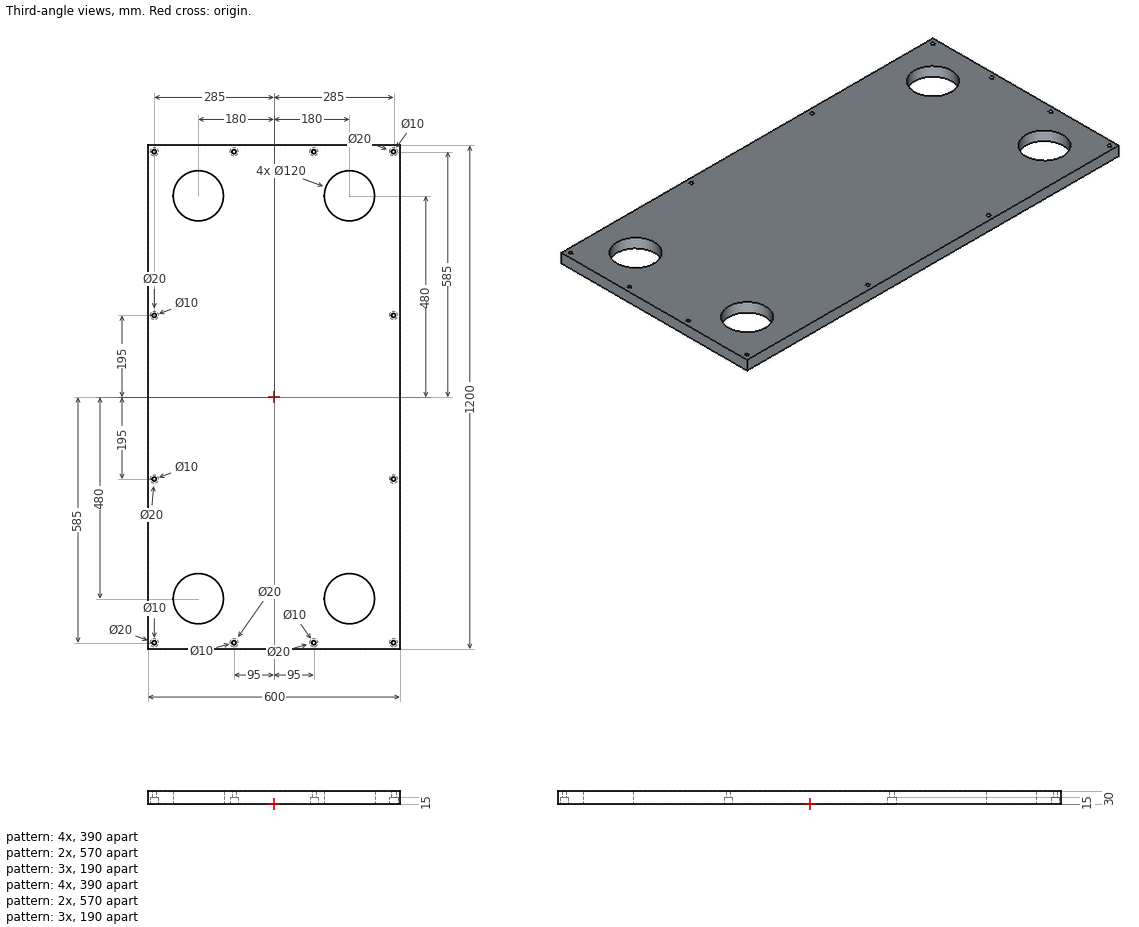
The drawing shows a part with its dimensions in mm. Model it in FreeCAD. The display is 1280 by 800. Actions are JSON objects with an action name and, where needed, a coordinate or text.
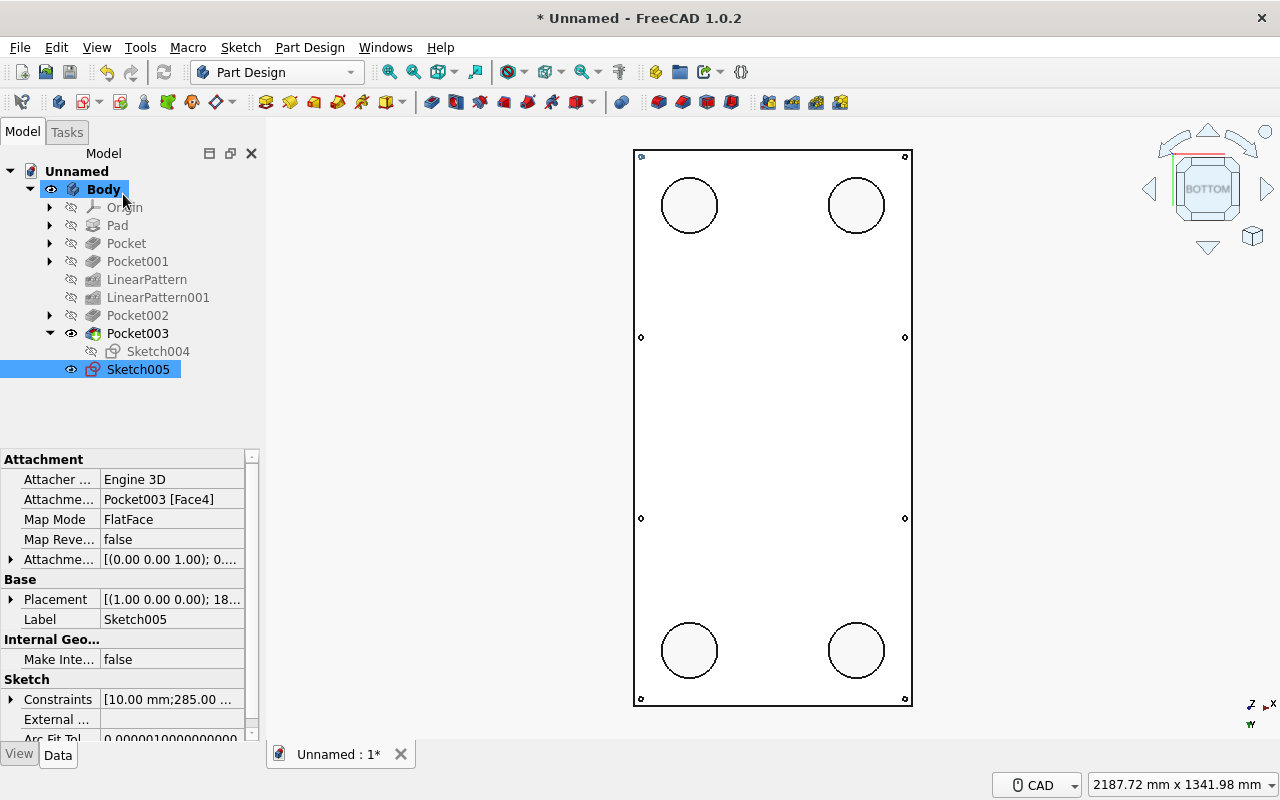
{"action": "left_click", "coordinate": [432, 102]}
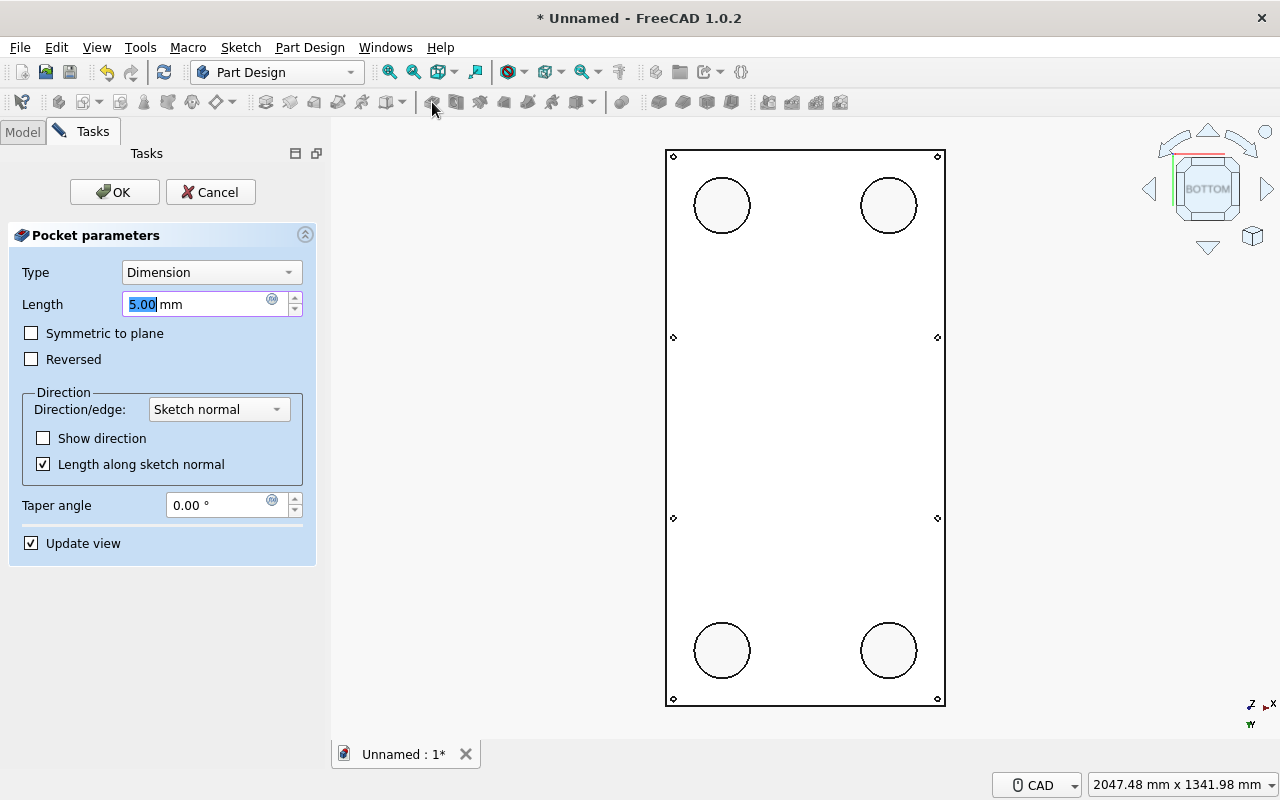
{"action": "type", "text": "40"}
{"action": "key", "text": "Tab"}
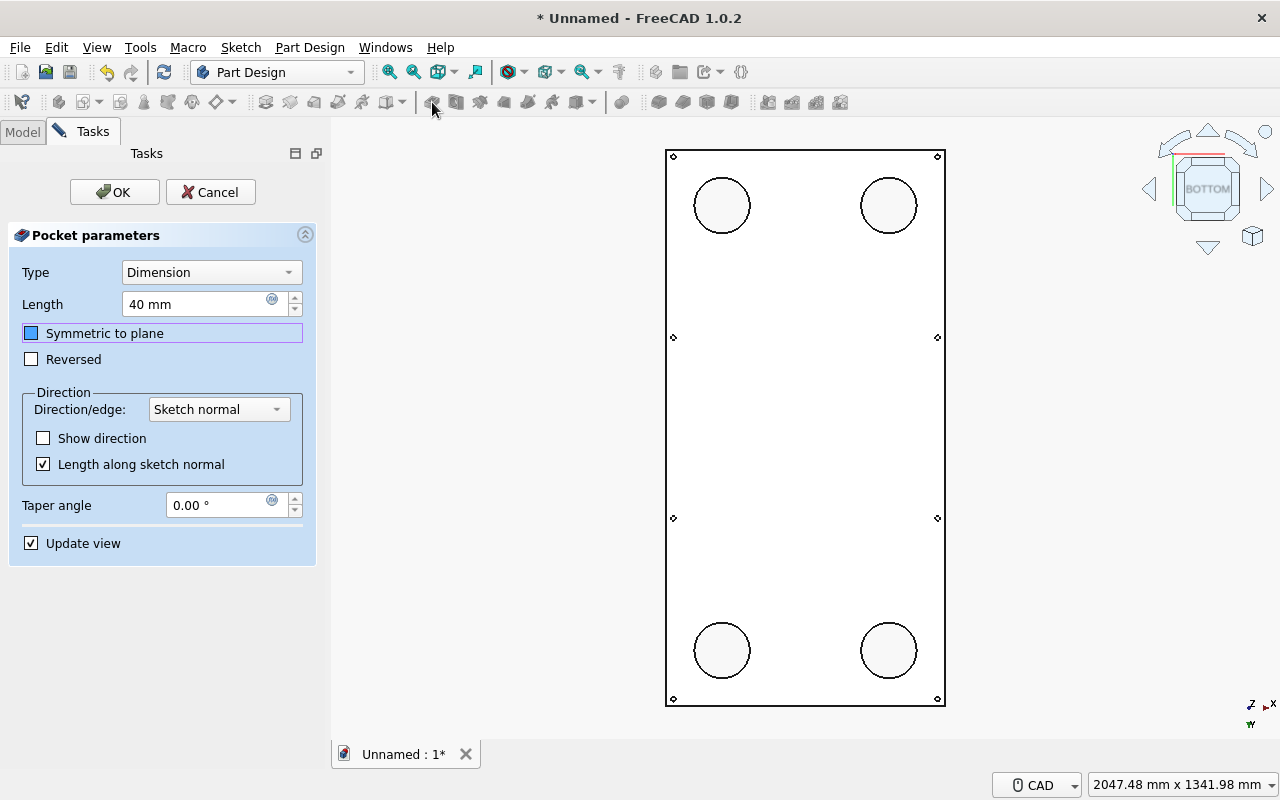
{"action": "left_click", "coordinate": [115, 192]}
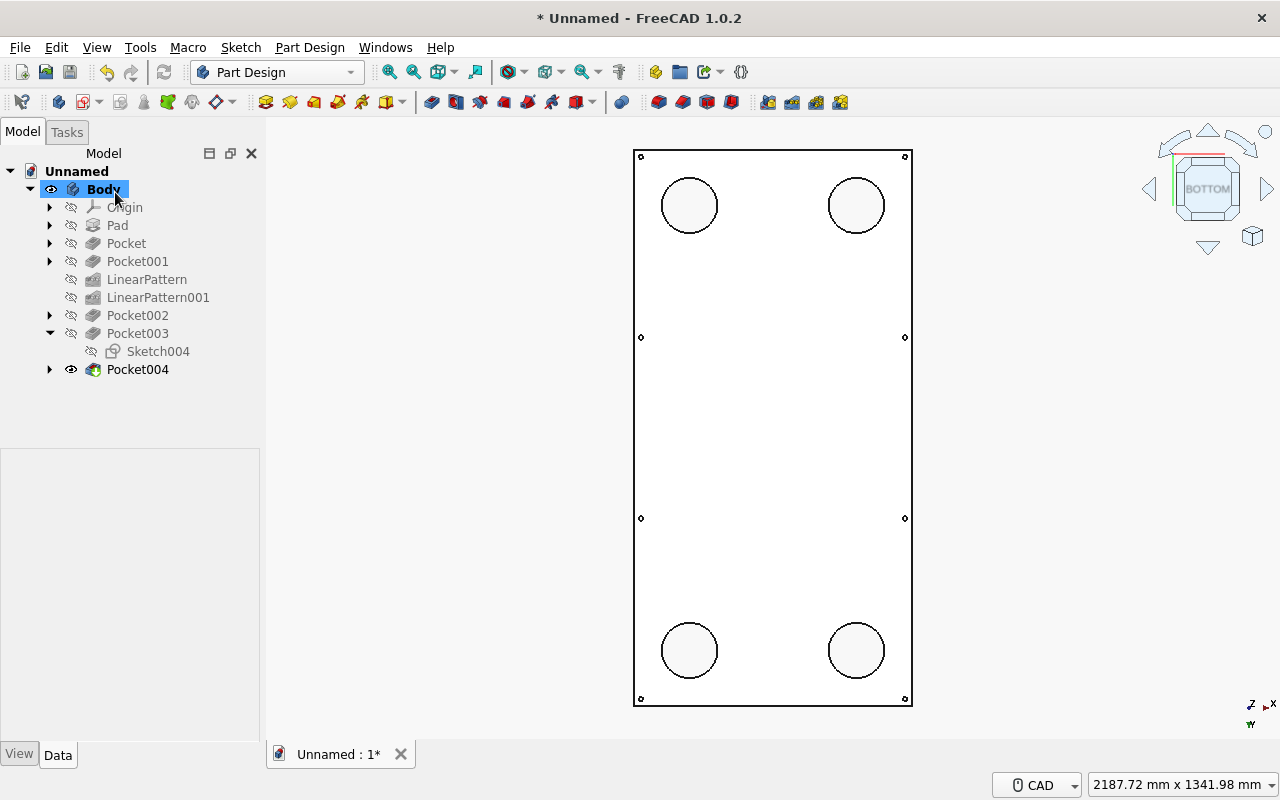
{"action": "left_click", "coordinate": [116, 261]}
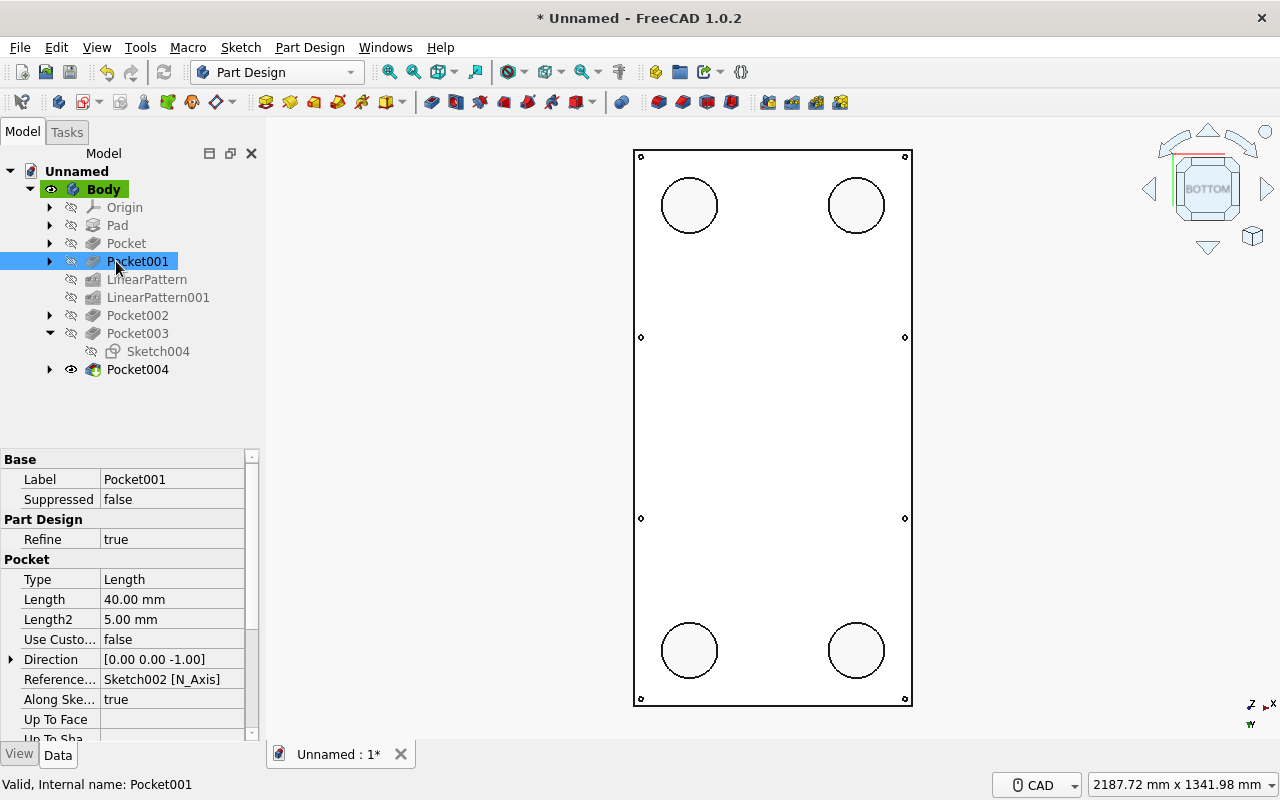
{"action": "left_click", "coordinate": [792, 102]}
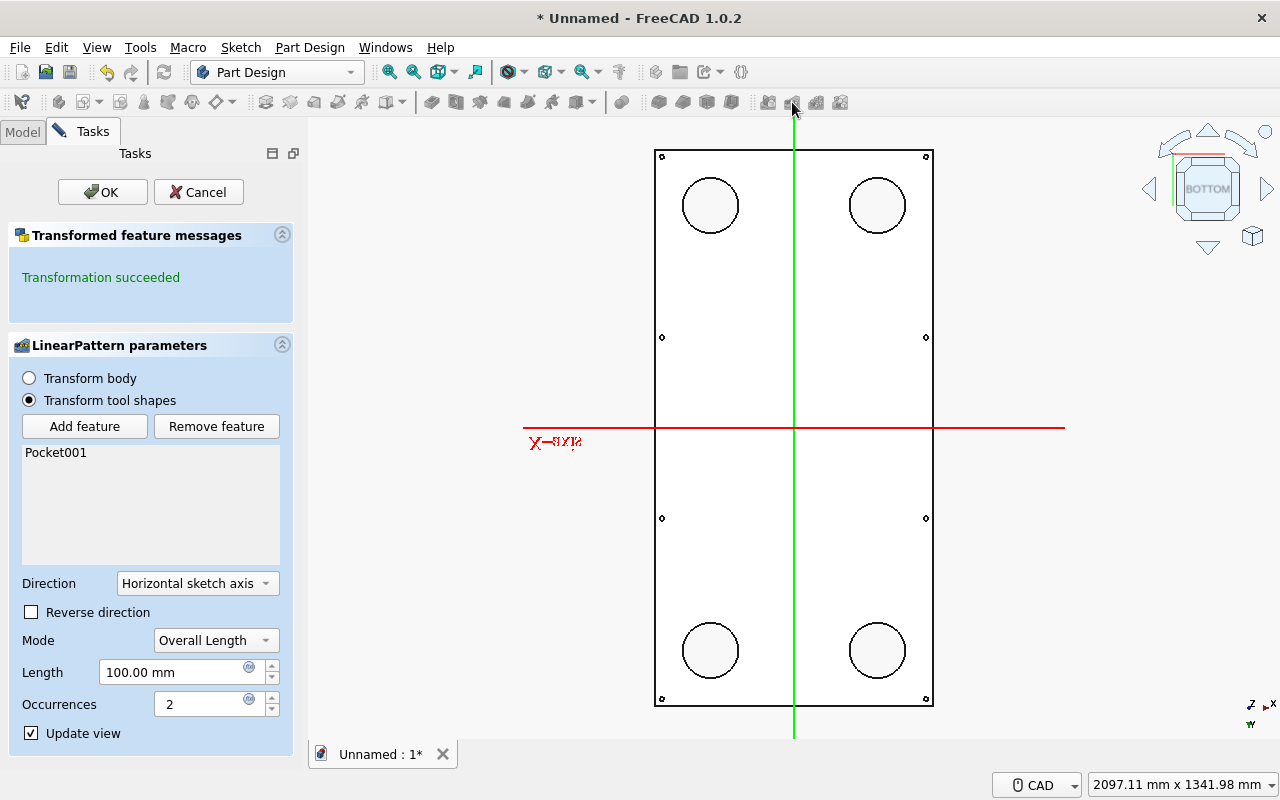
{"action": "left_click", "coordinate": [198, 584]}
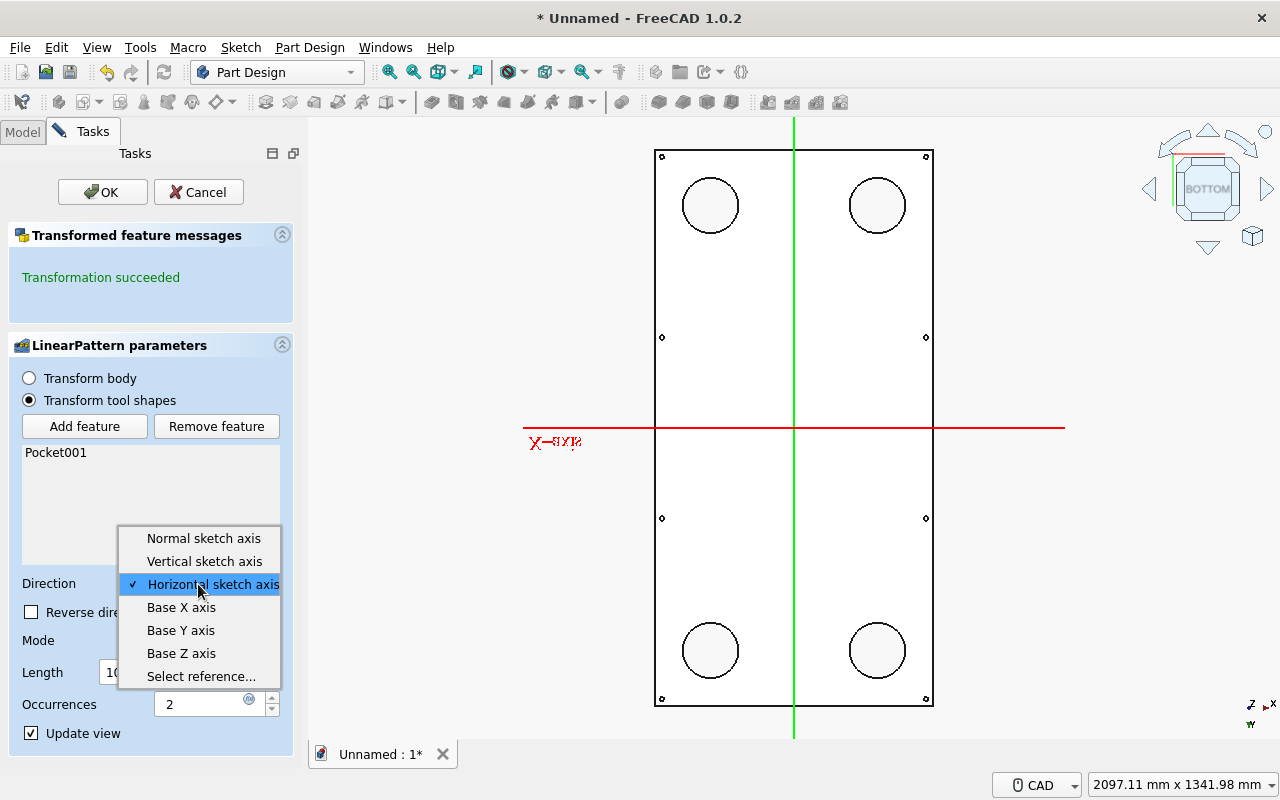
{"action": "left_click", "coordinate": [198, 608]}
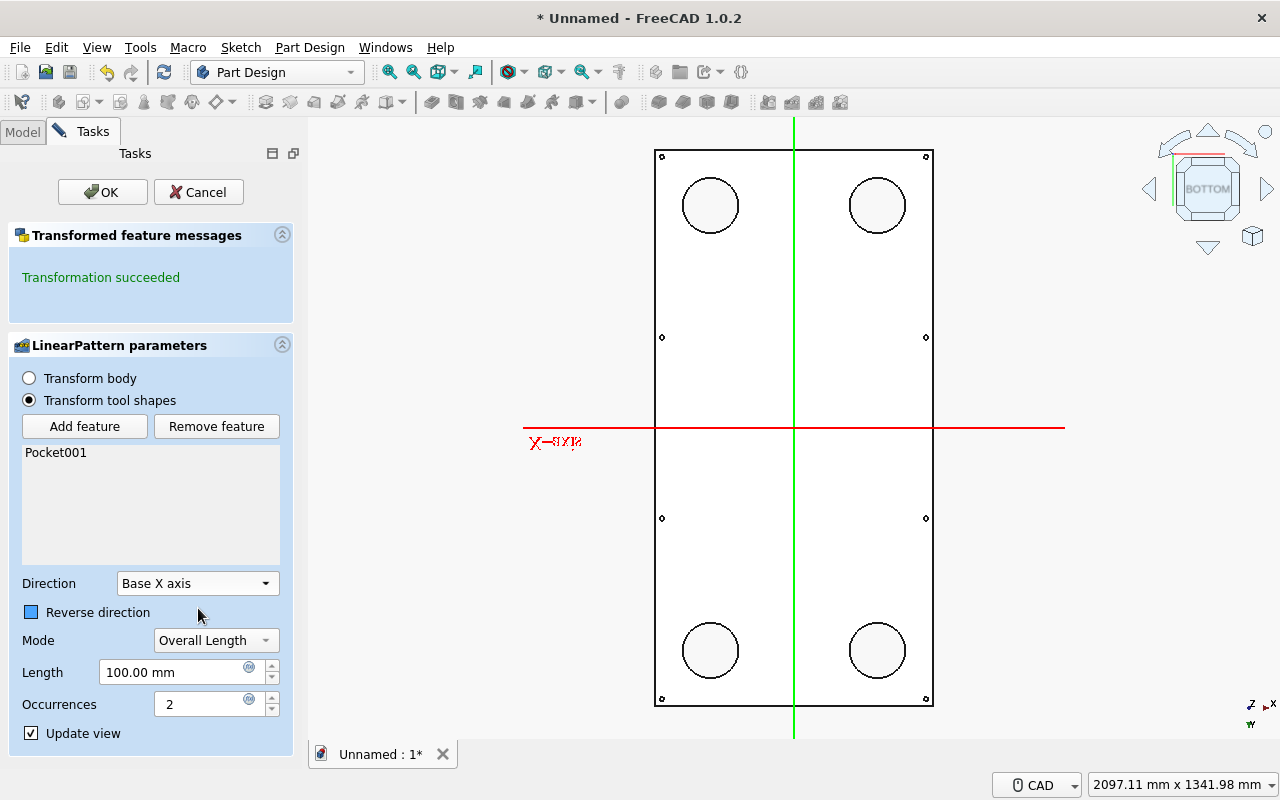
{"action": "left_click", "coordinate": [217, 640]}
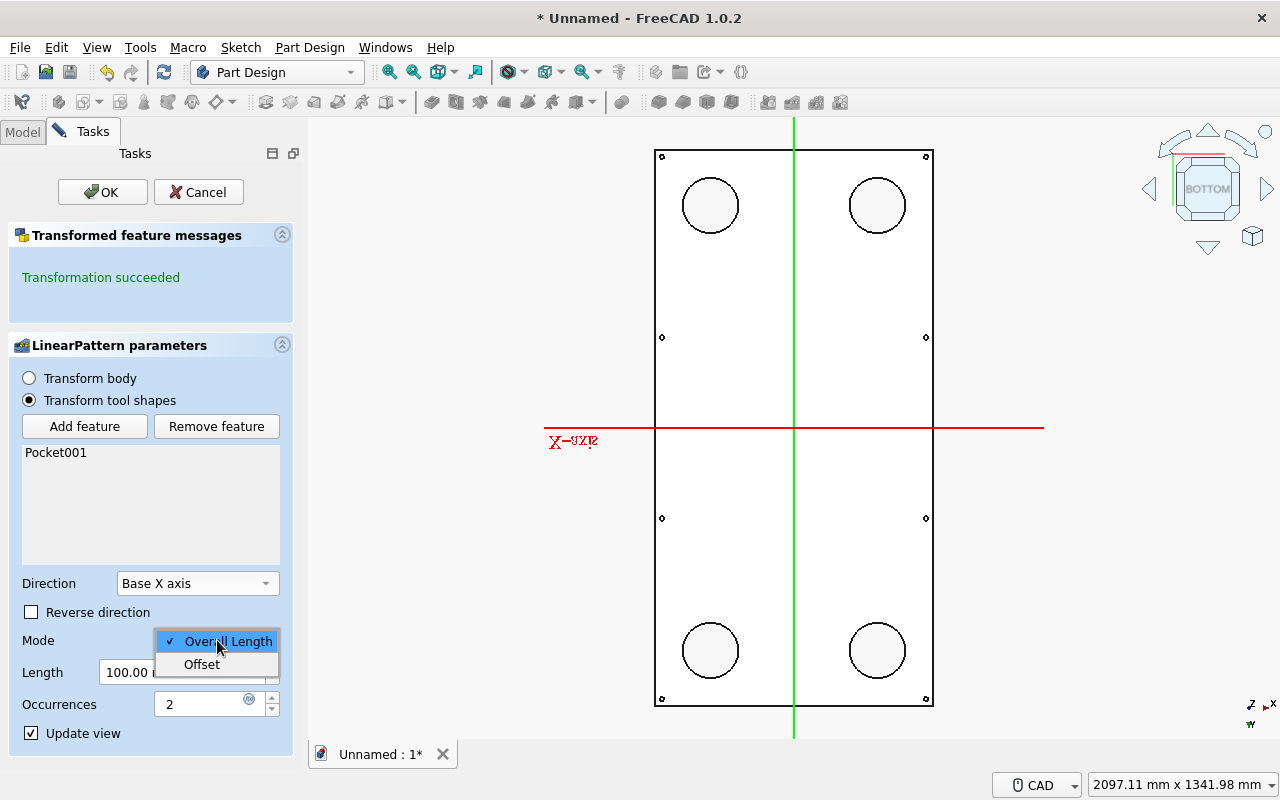
{"action": "left_click", "coordinate": [216, 664]}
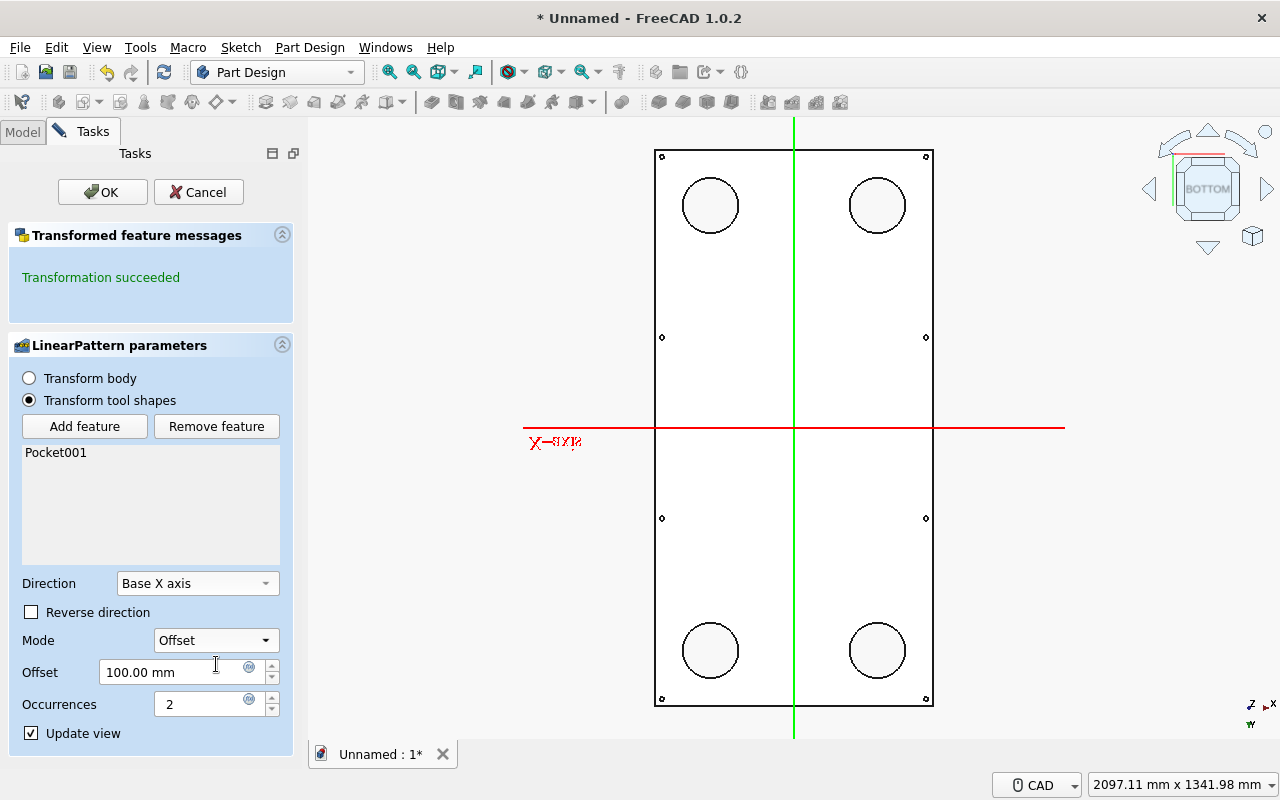
{"action": "triple_click", "coordinate": [182, 672]}